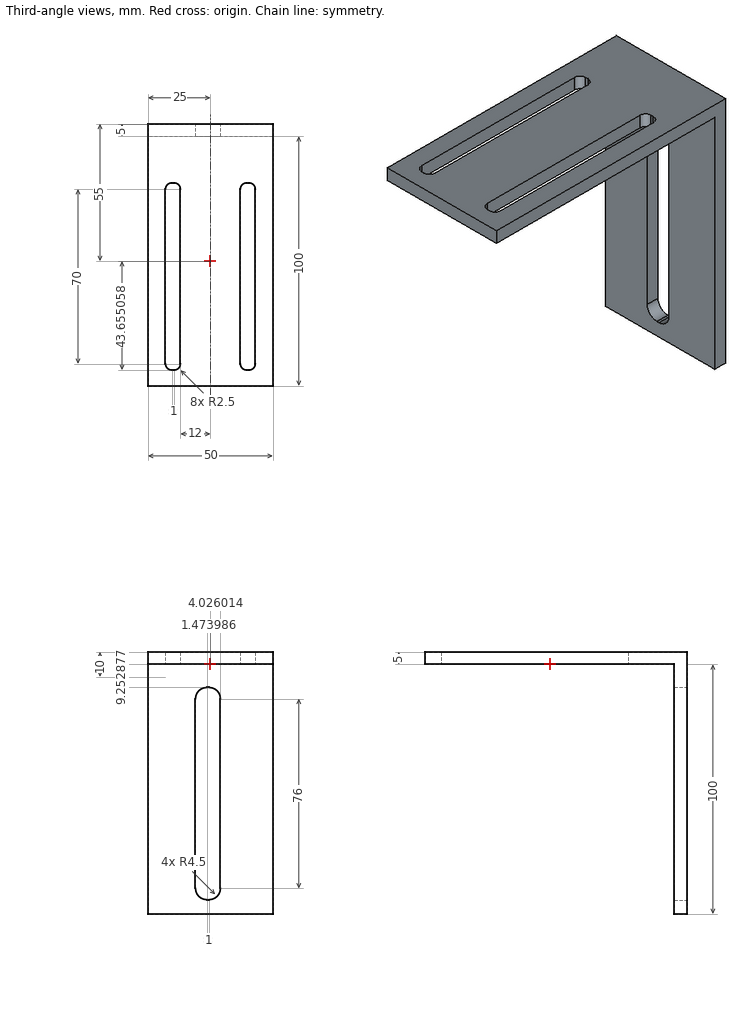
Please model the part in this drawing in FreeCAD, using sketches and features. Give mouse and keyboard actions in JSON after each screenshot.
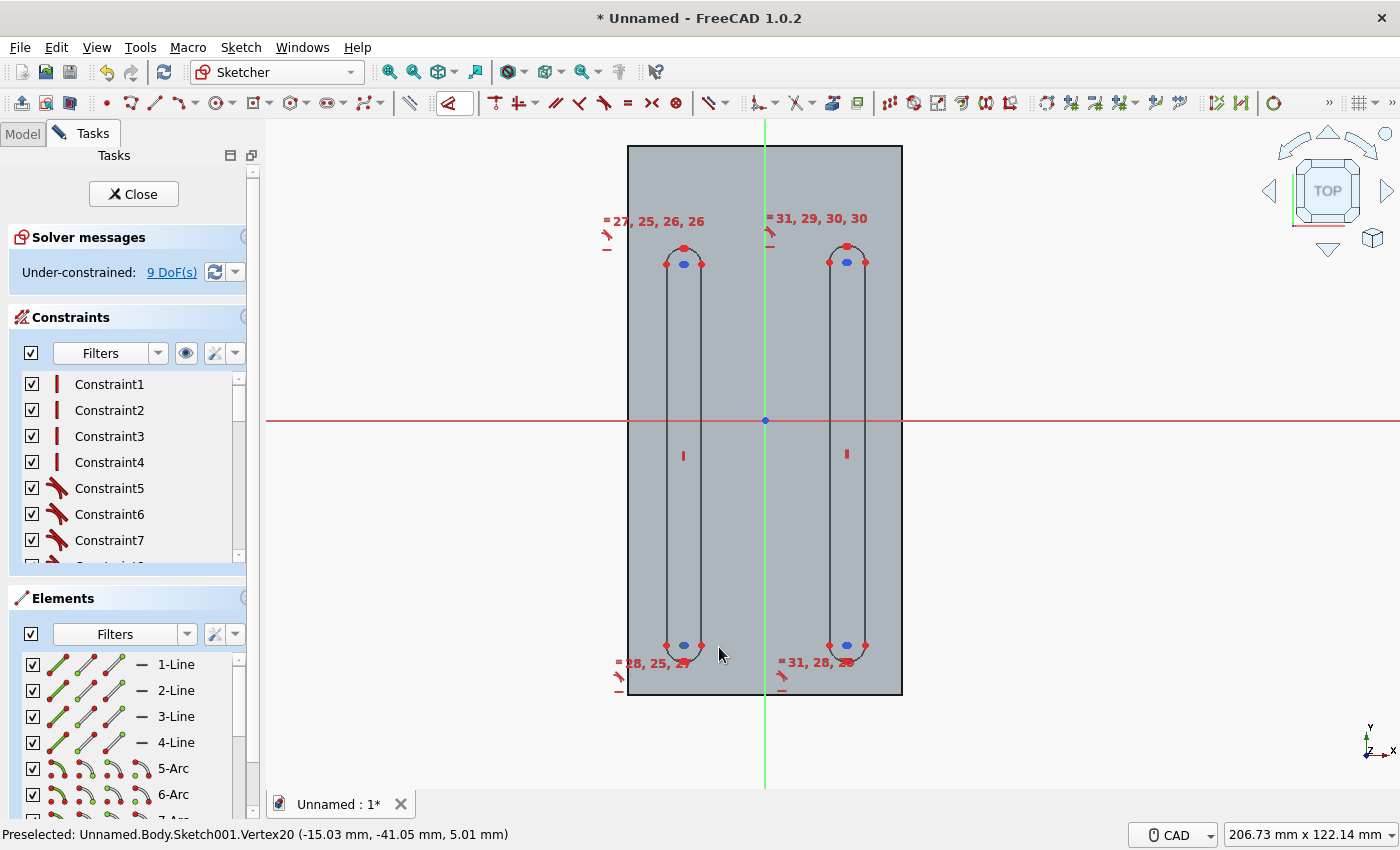
{"action": "scroll", "coordinate": [849, 645], "scroll_direction": "up", "scroll_amount": 7}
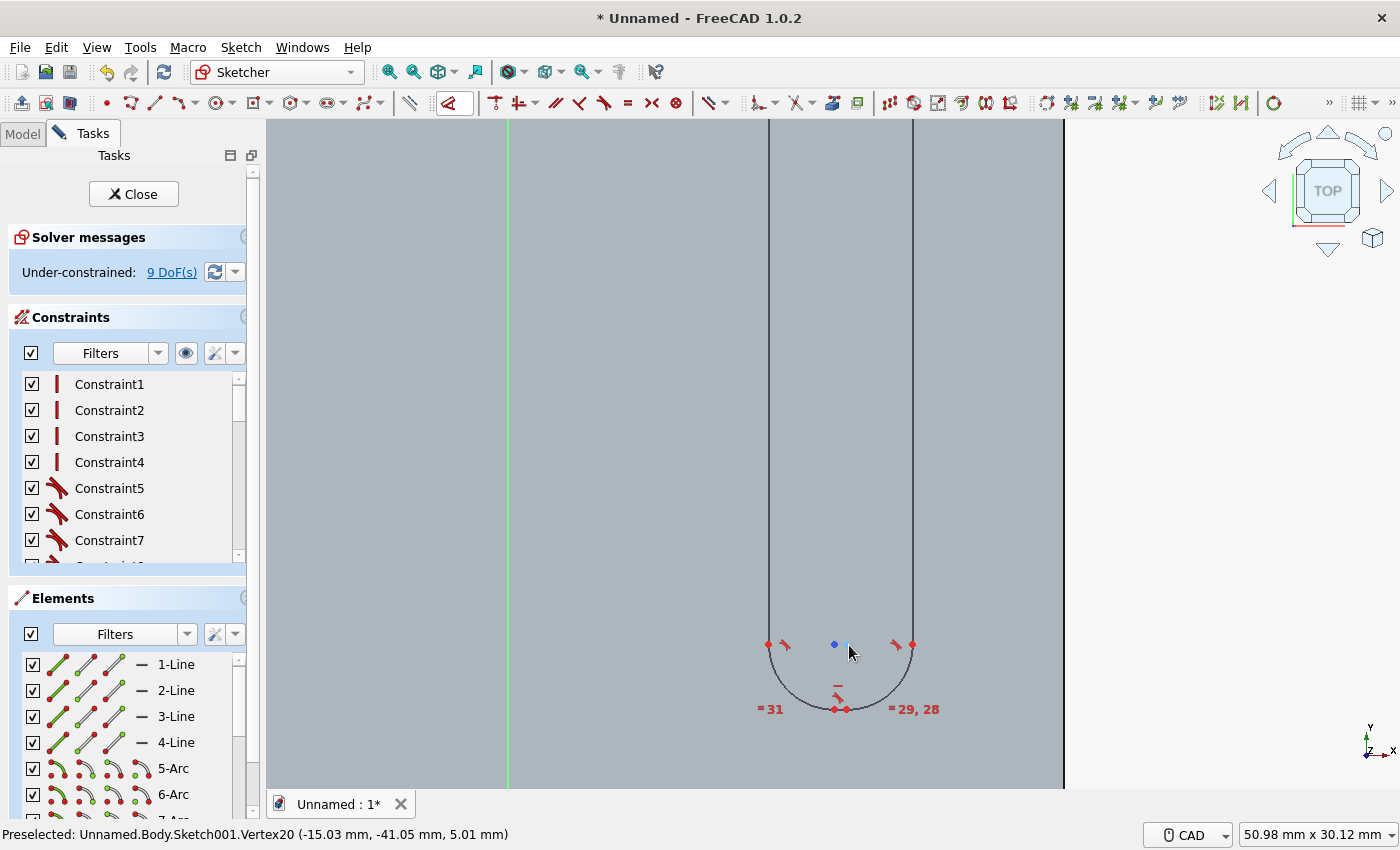
{"action": "left_click", "coordinate": [847, 644]}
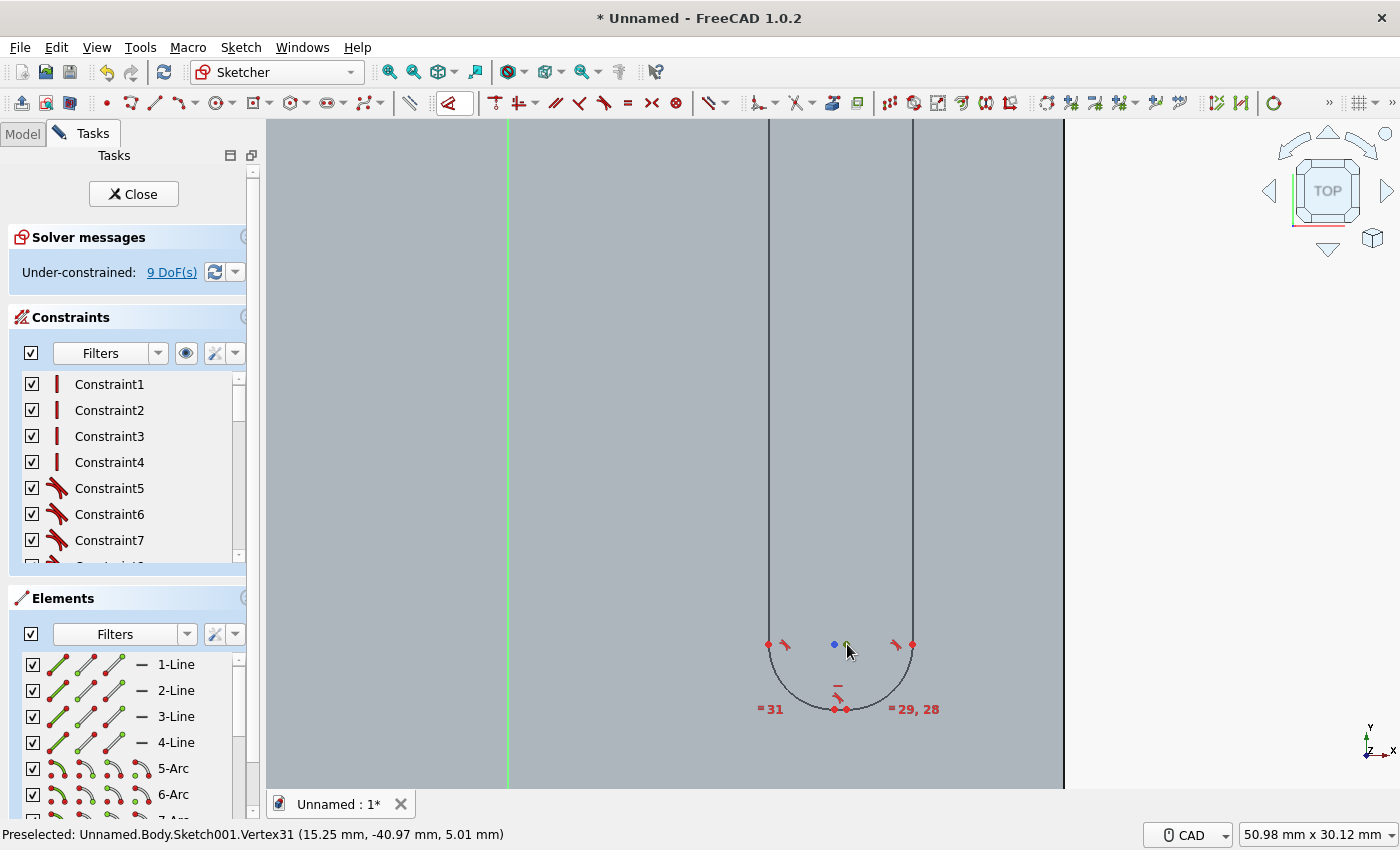
{"action": "left_click", "coordinate": [508, 717]}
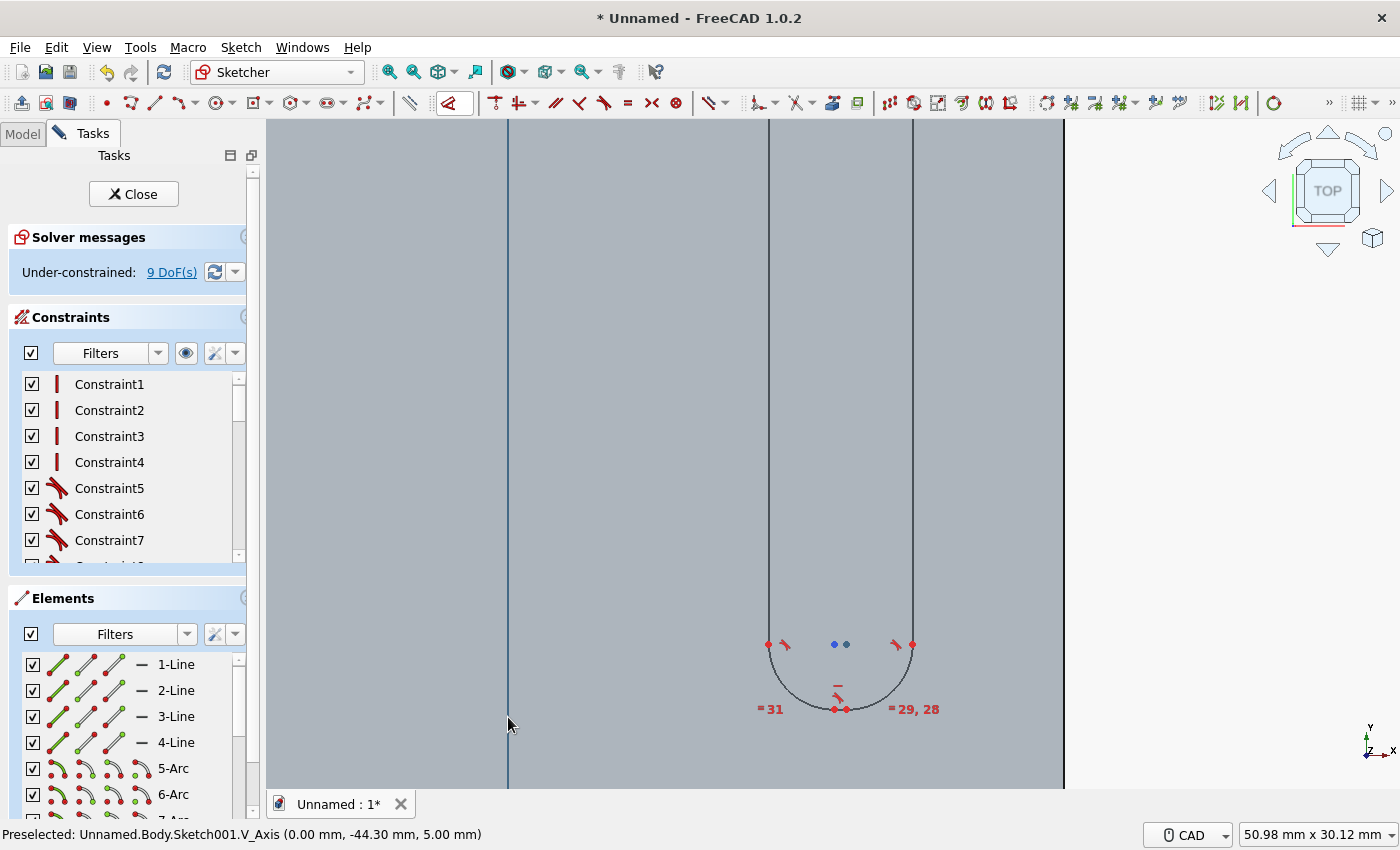
{"action": "left_click", "coordinate": [652, 104]}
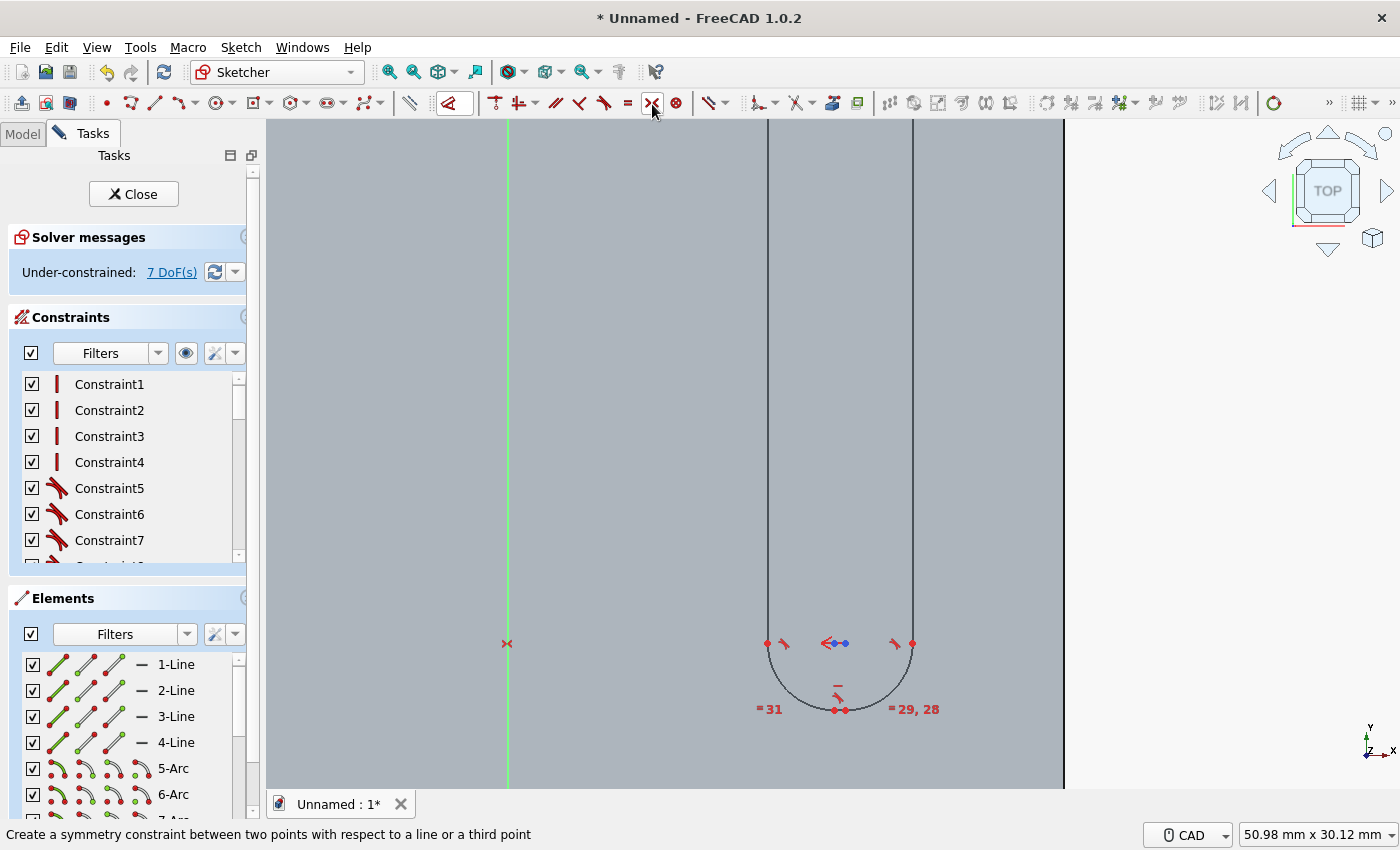
{"action": "scroll", "coordinate": [849, 645], "scroll_direction": "down", "scroll_amount": 7}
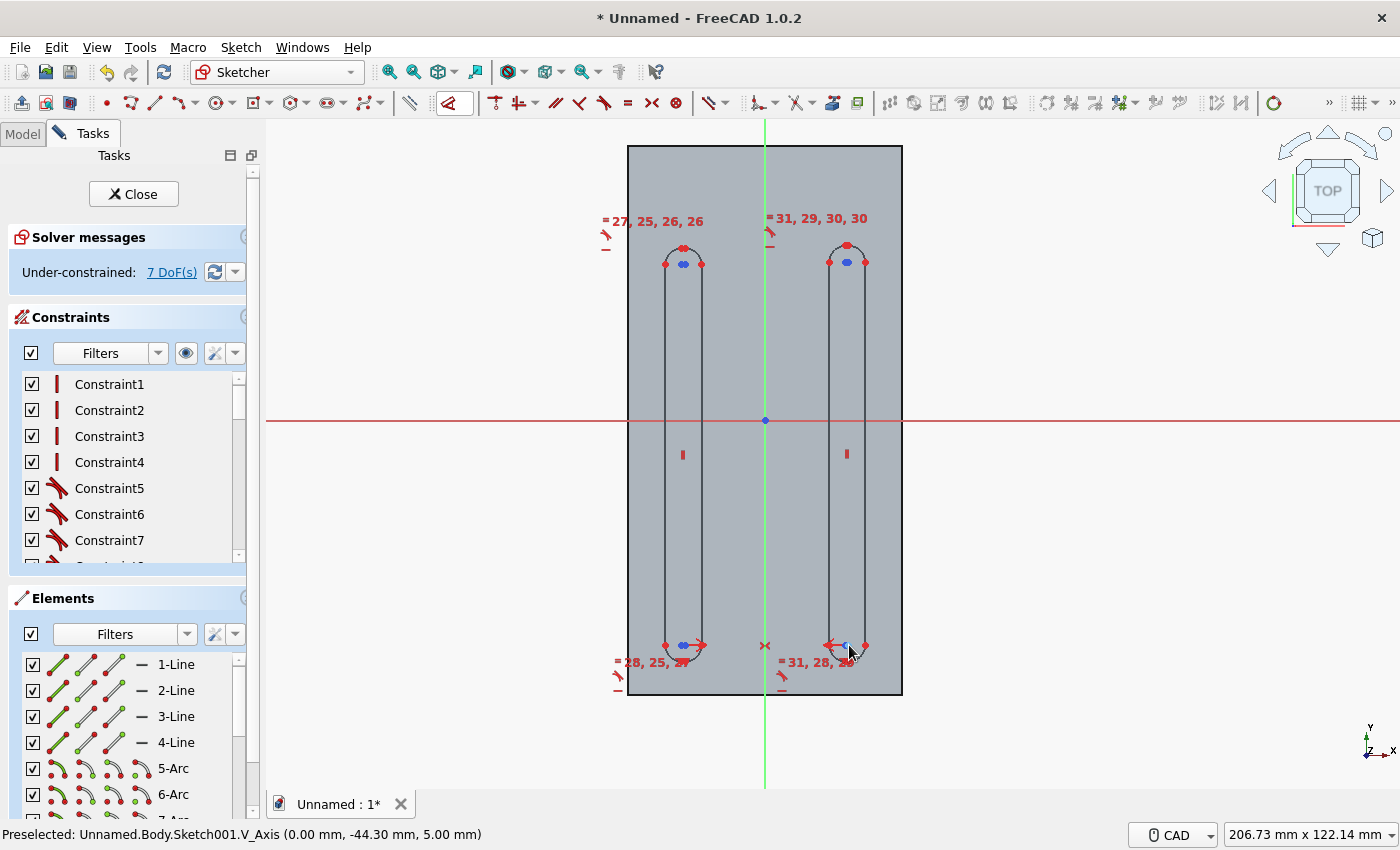
{"action": "scroll", "coordinate": [685, 265], "scroll_direction": "up", "scroll_amount": 7}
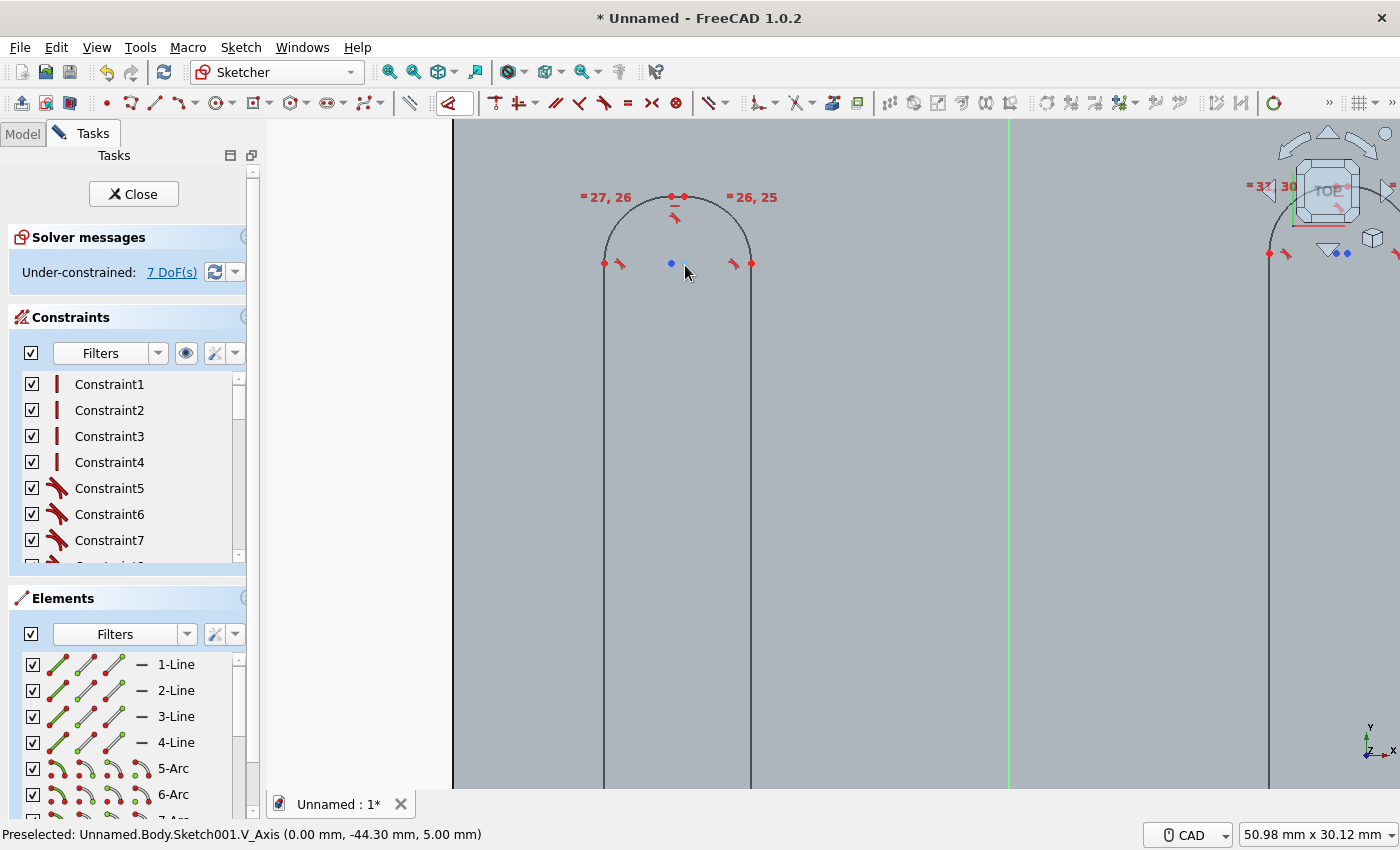
{"action": "left_click", "coordinate": [684, 263]}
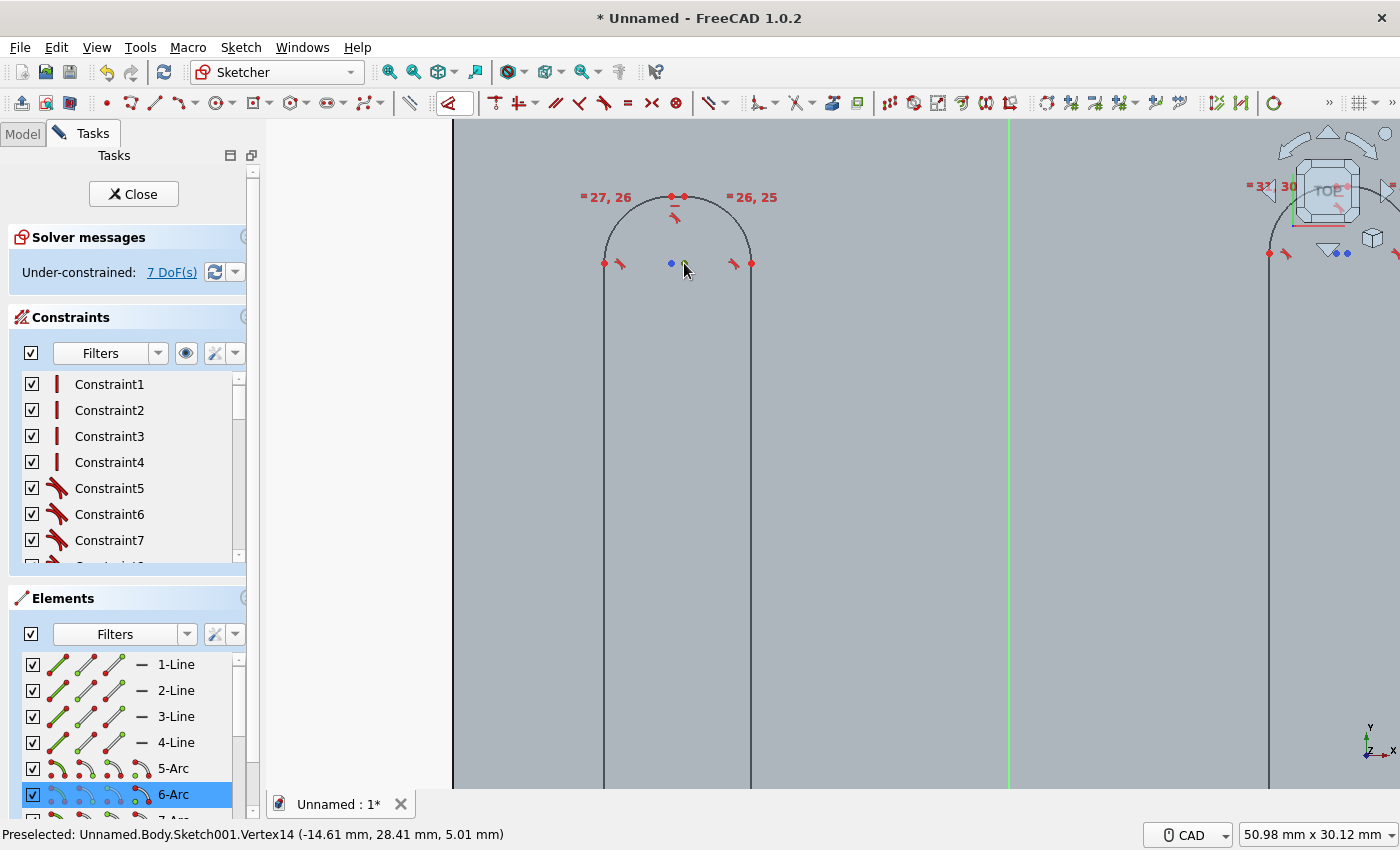
{"action": "scroll", "coordinate": [684, 265], "scroll_direction": "down", "scroll_amount": 7}